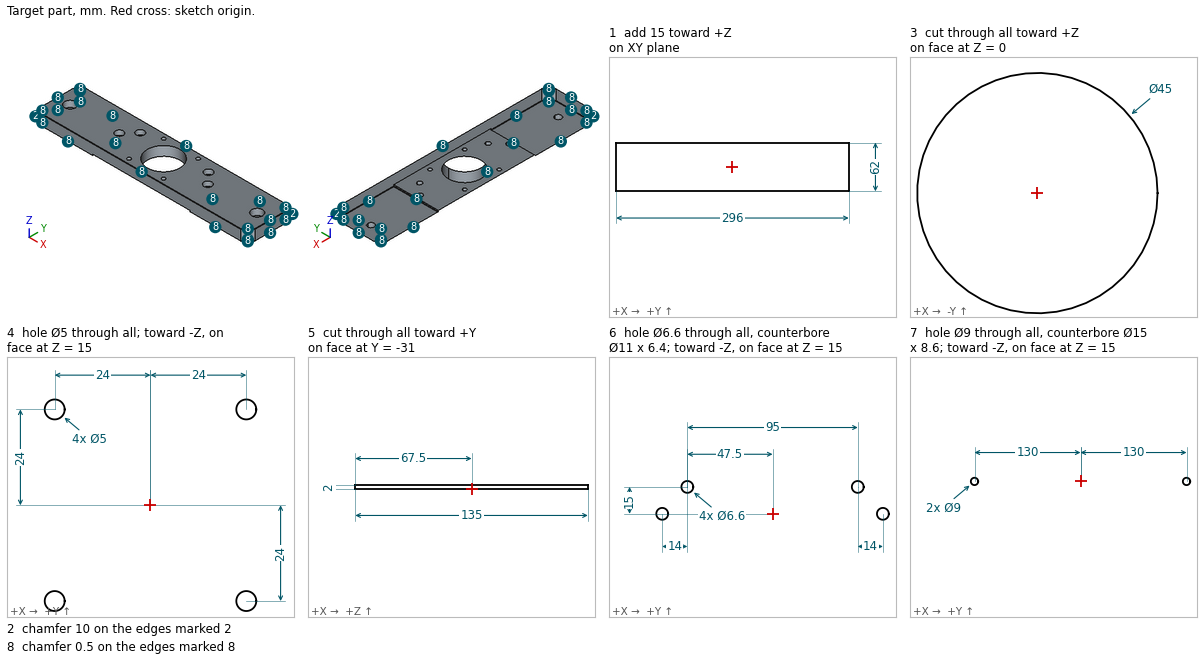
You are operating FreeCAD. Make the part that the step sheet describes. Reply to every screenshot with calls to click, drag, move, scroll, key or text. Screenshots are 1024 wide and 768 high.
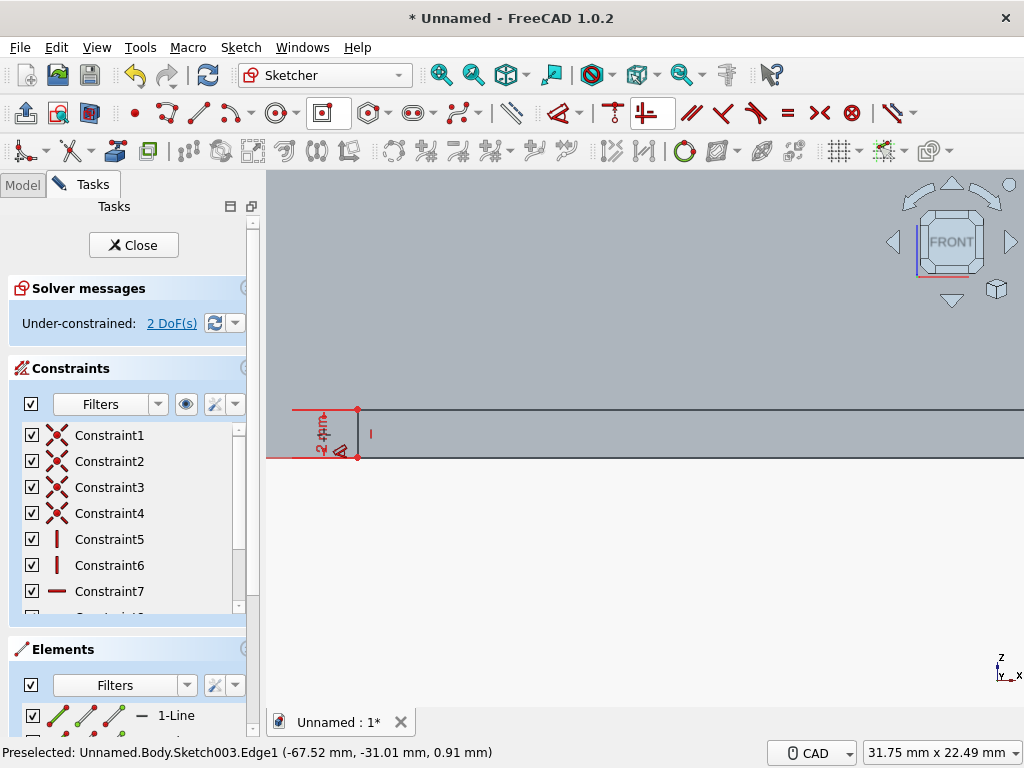
scroll(358, 439, down, 10)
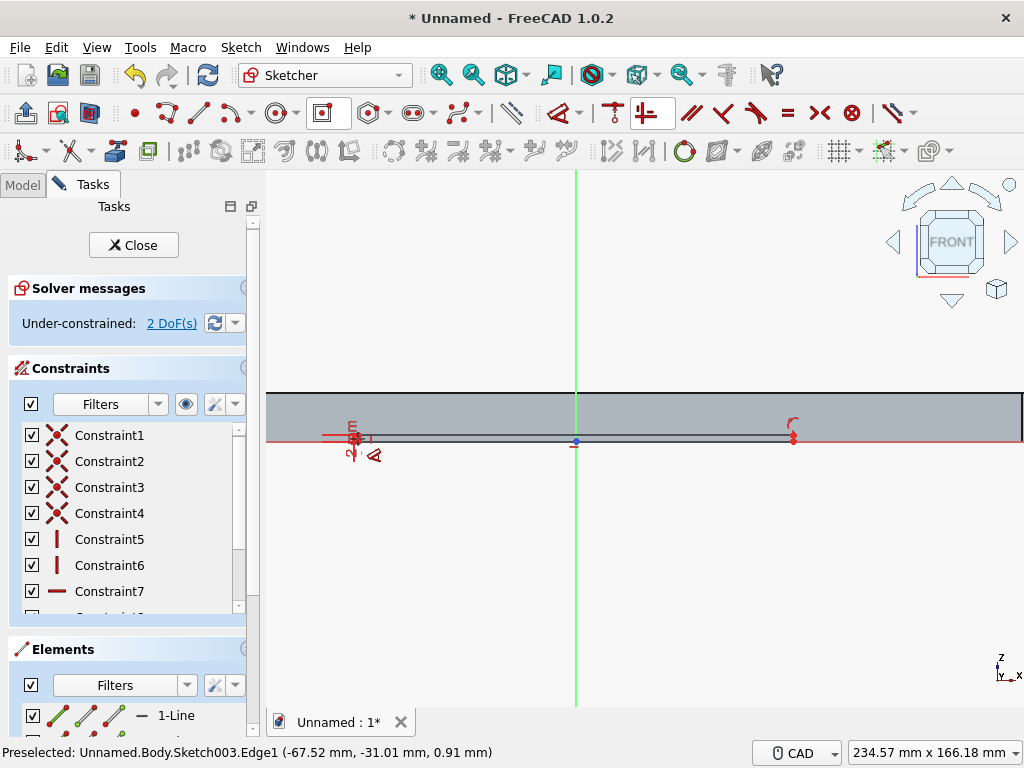
scroll(489, 442, up, 4)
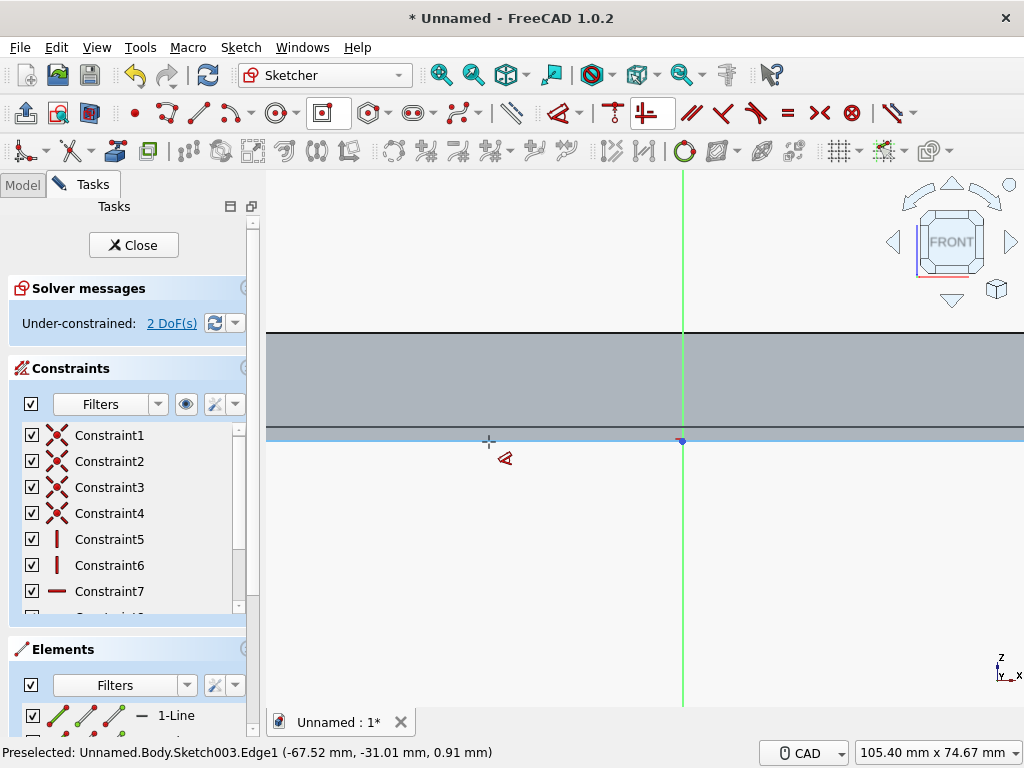
click(488, 441)
click(576, 475)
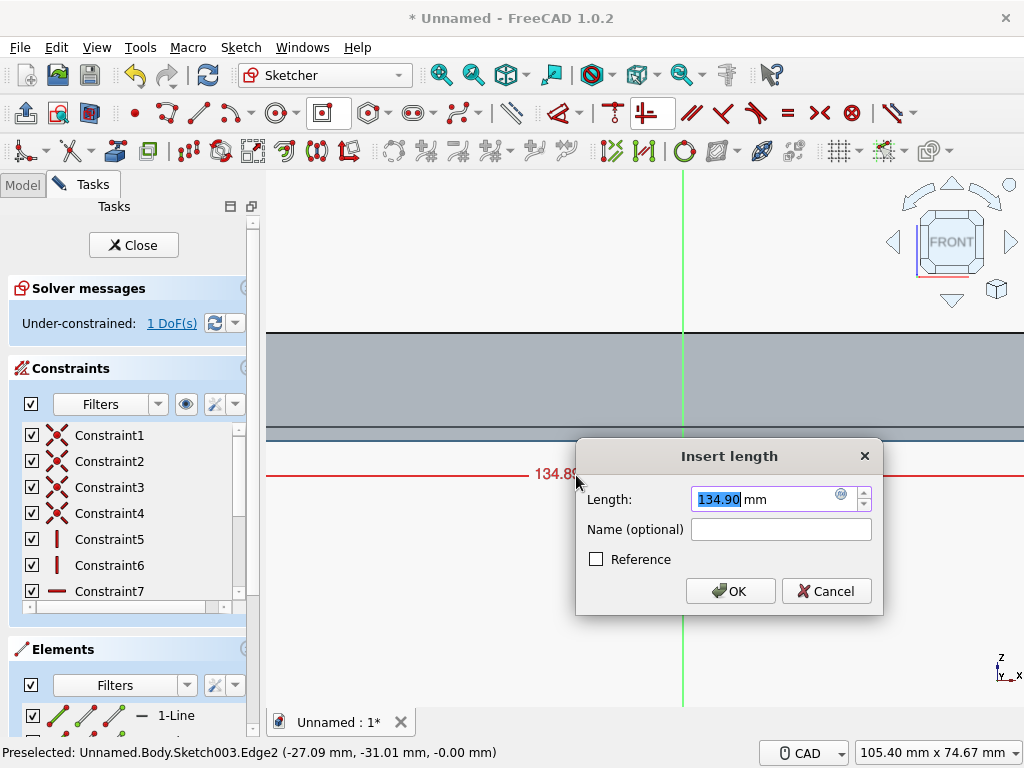
text(135)
key(Return)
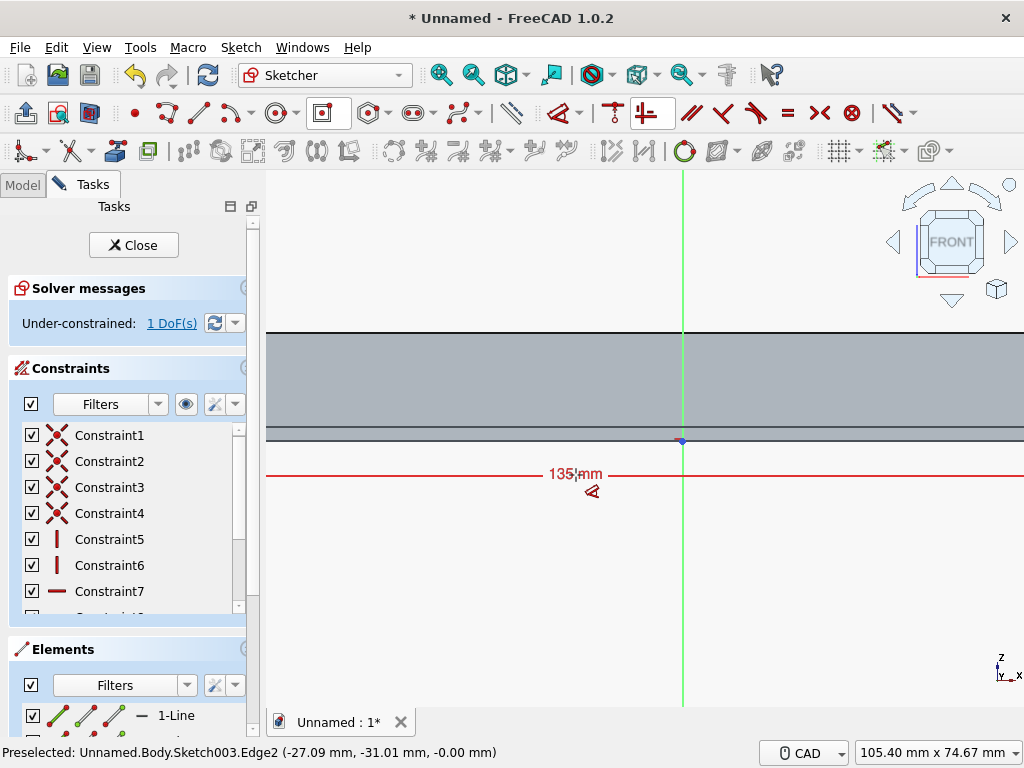
scroll(490, 442, down, 4)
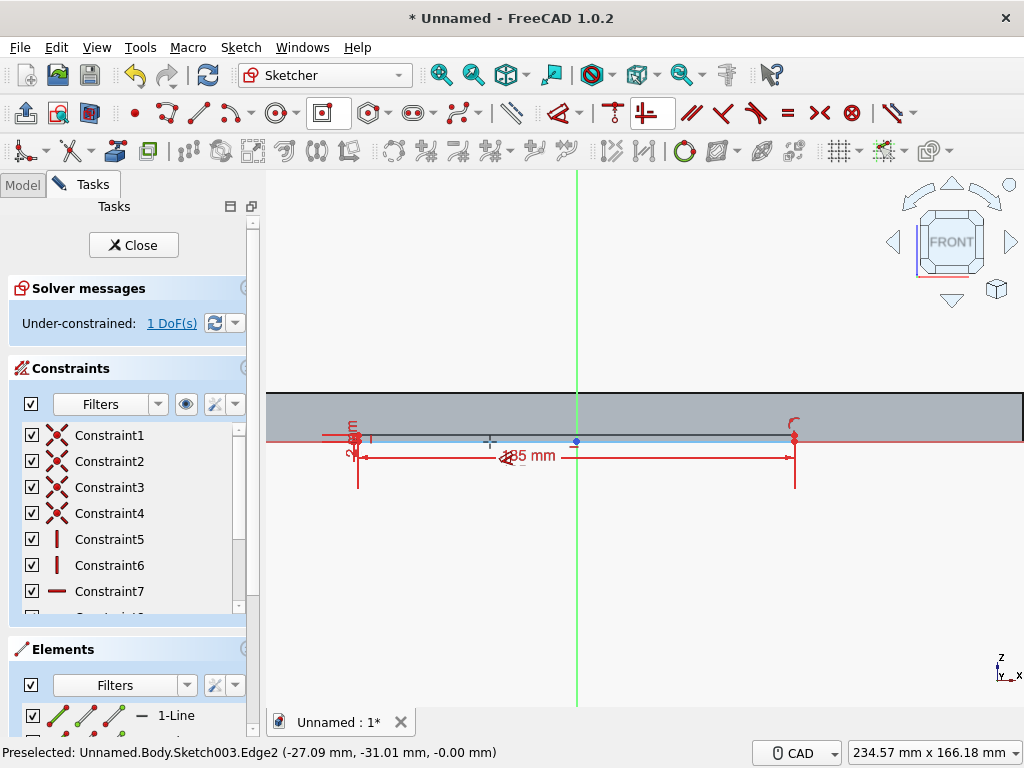
scroll(358, 435, up, 4)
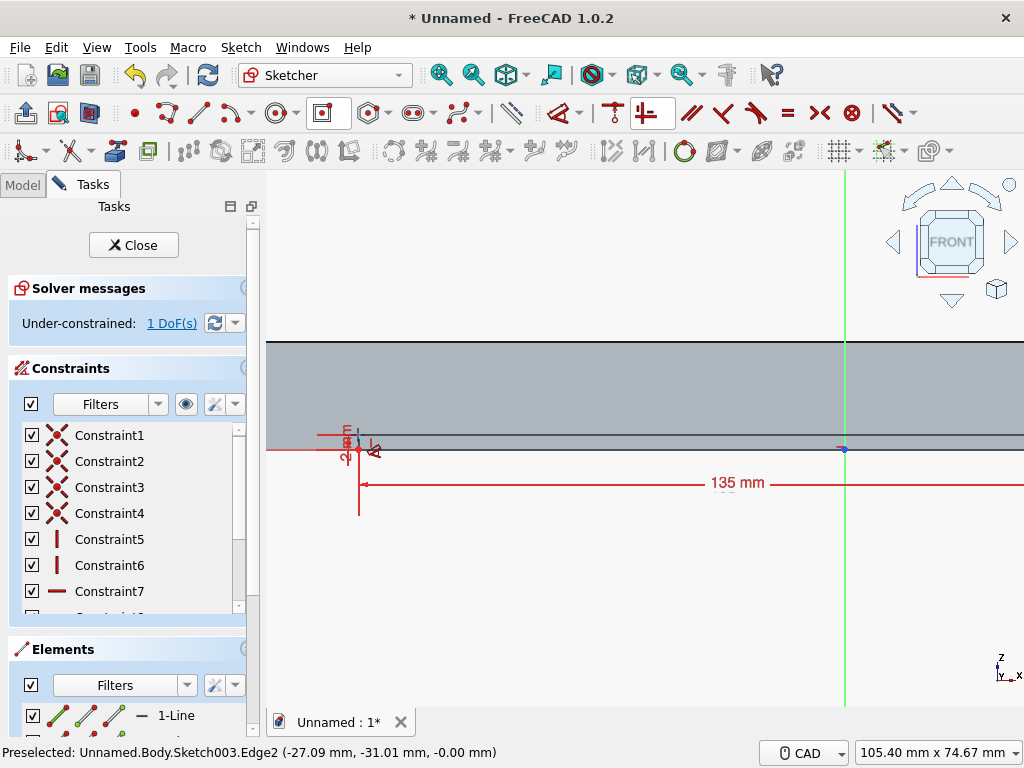
click(359, 435)
click(602, 484)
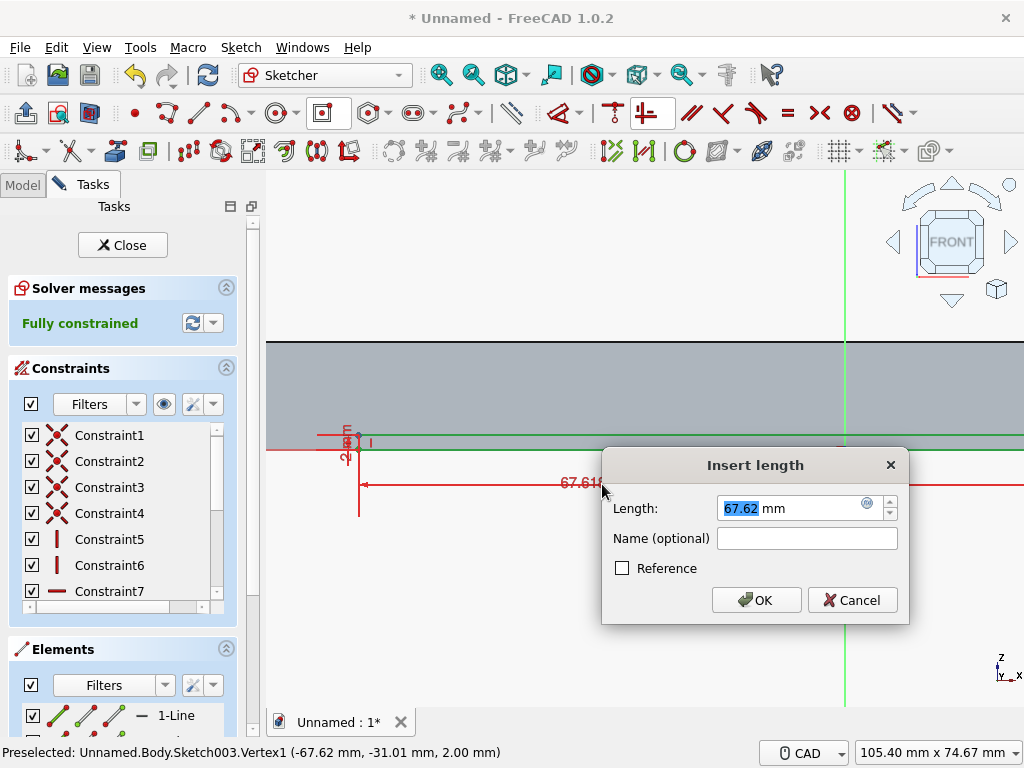
text(67.5)
key(Return)
key(Escape)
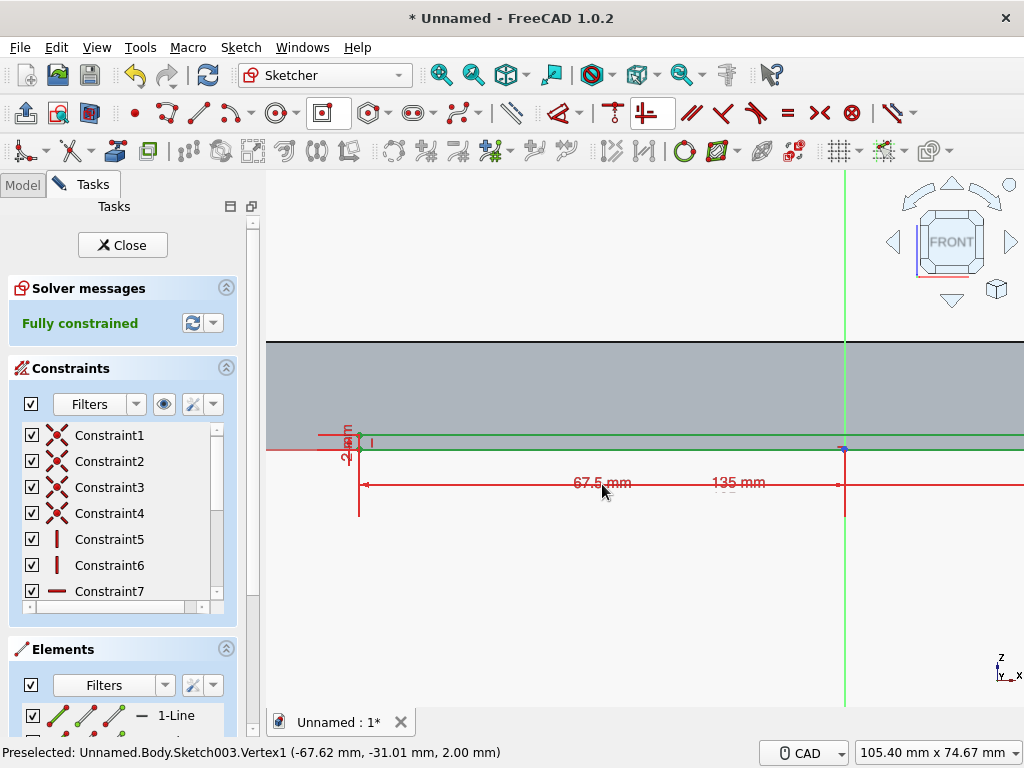
click(123, 245)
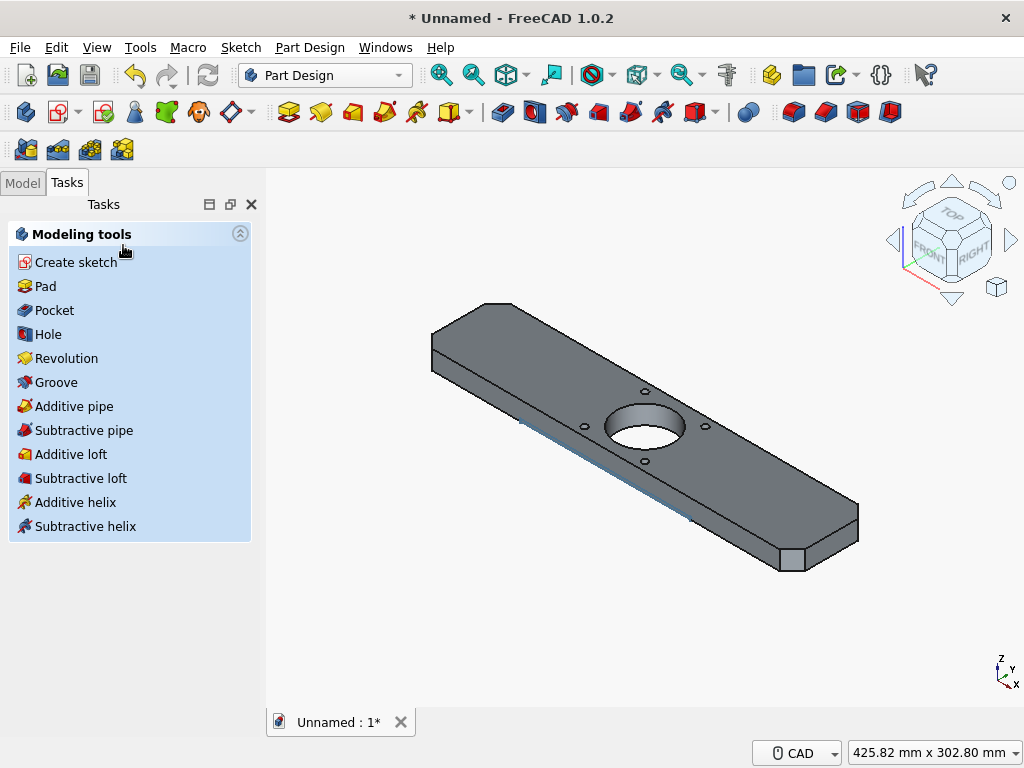
click(504, 112)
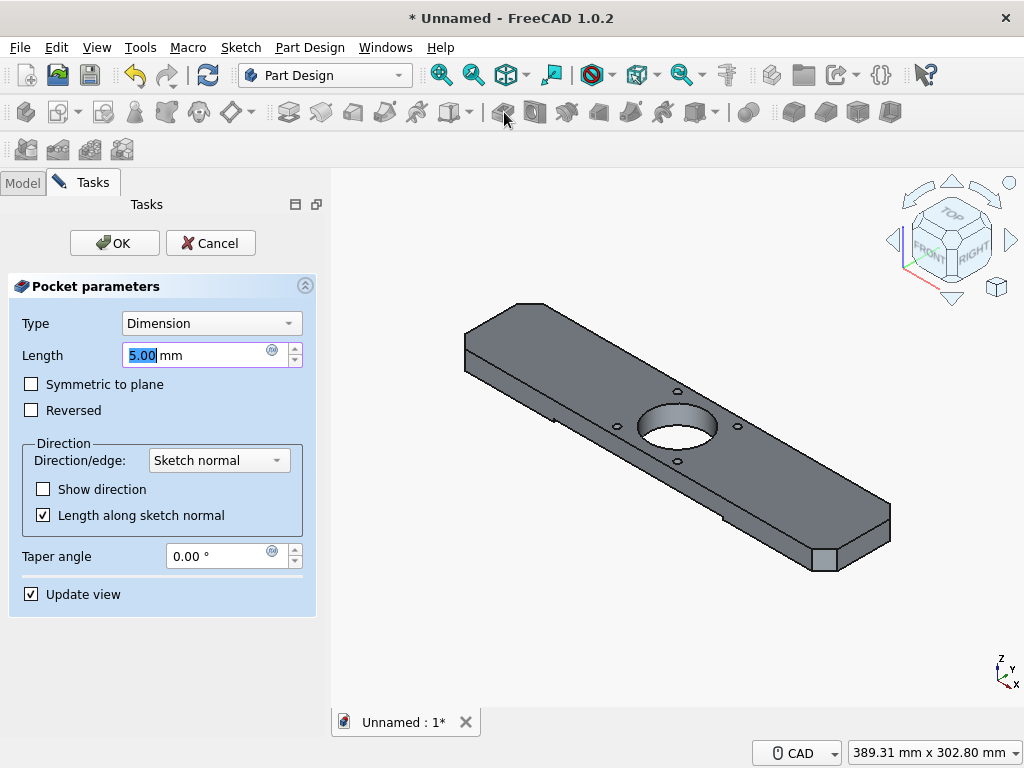
click(212, 324)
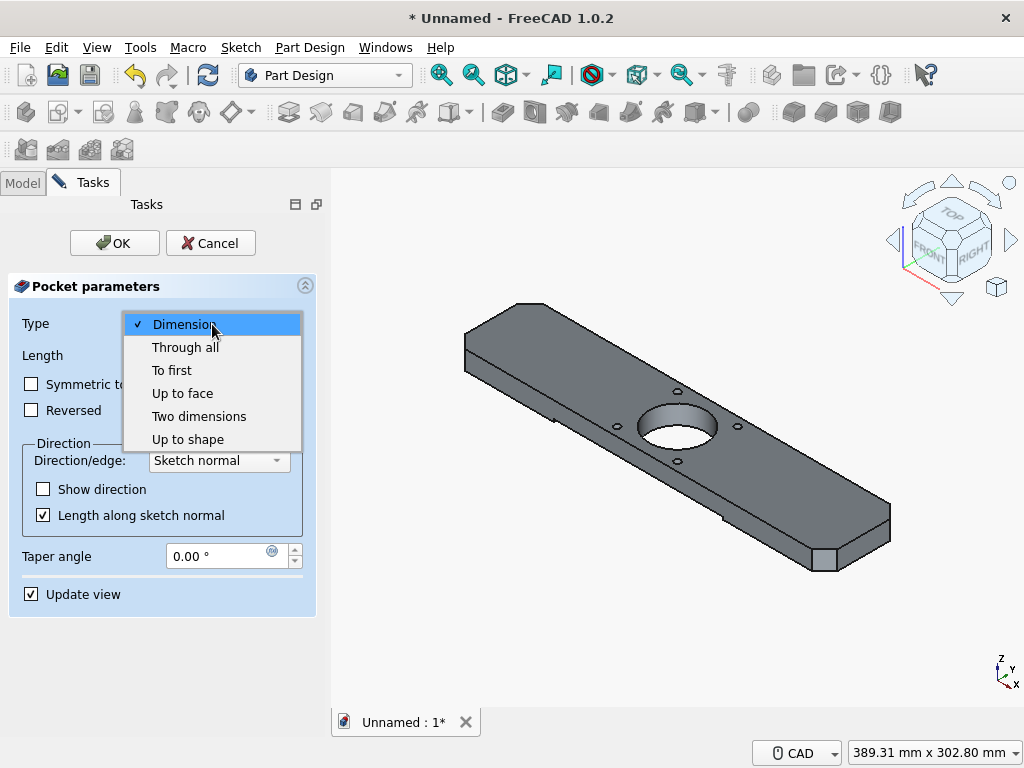
click(212, 348)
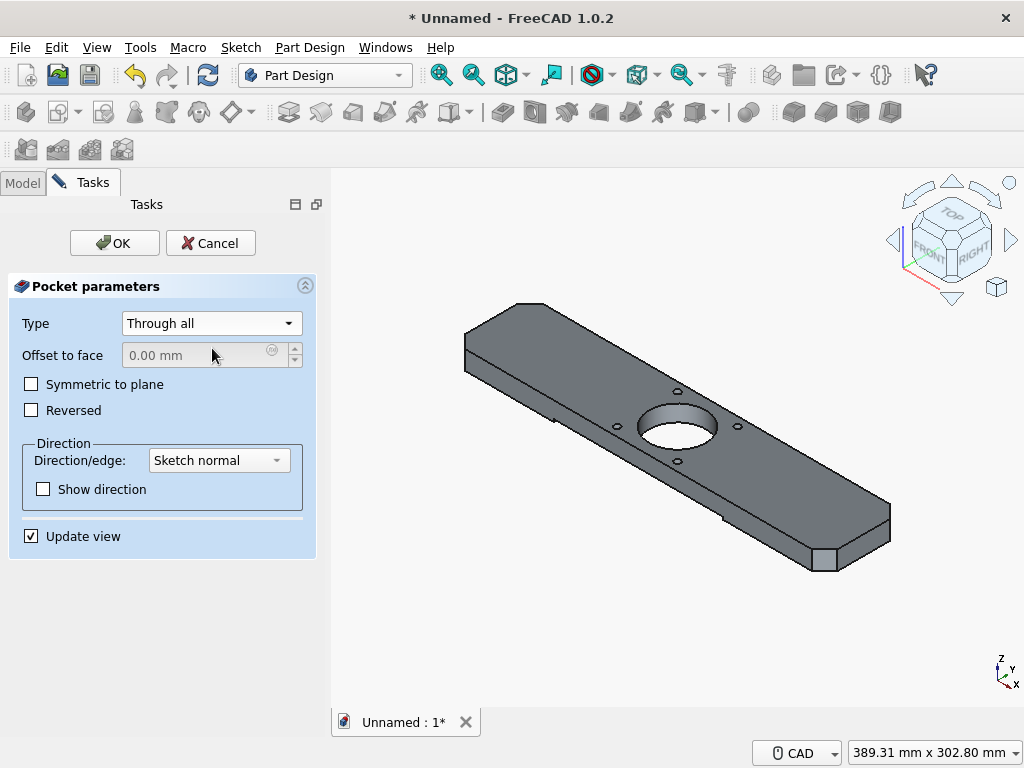
click(115, 243)